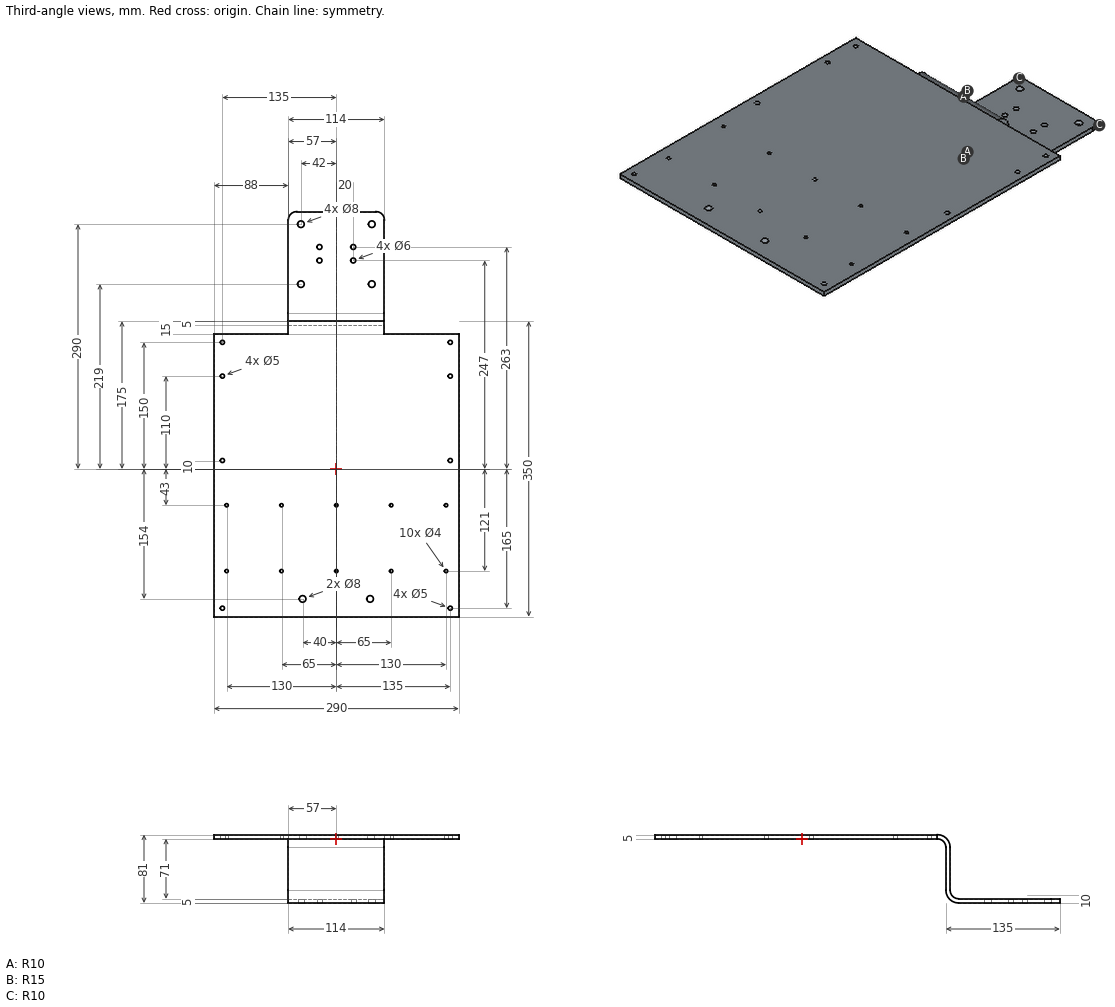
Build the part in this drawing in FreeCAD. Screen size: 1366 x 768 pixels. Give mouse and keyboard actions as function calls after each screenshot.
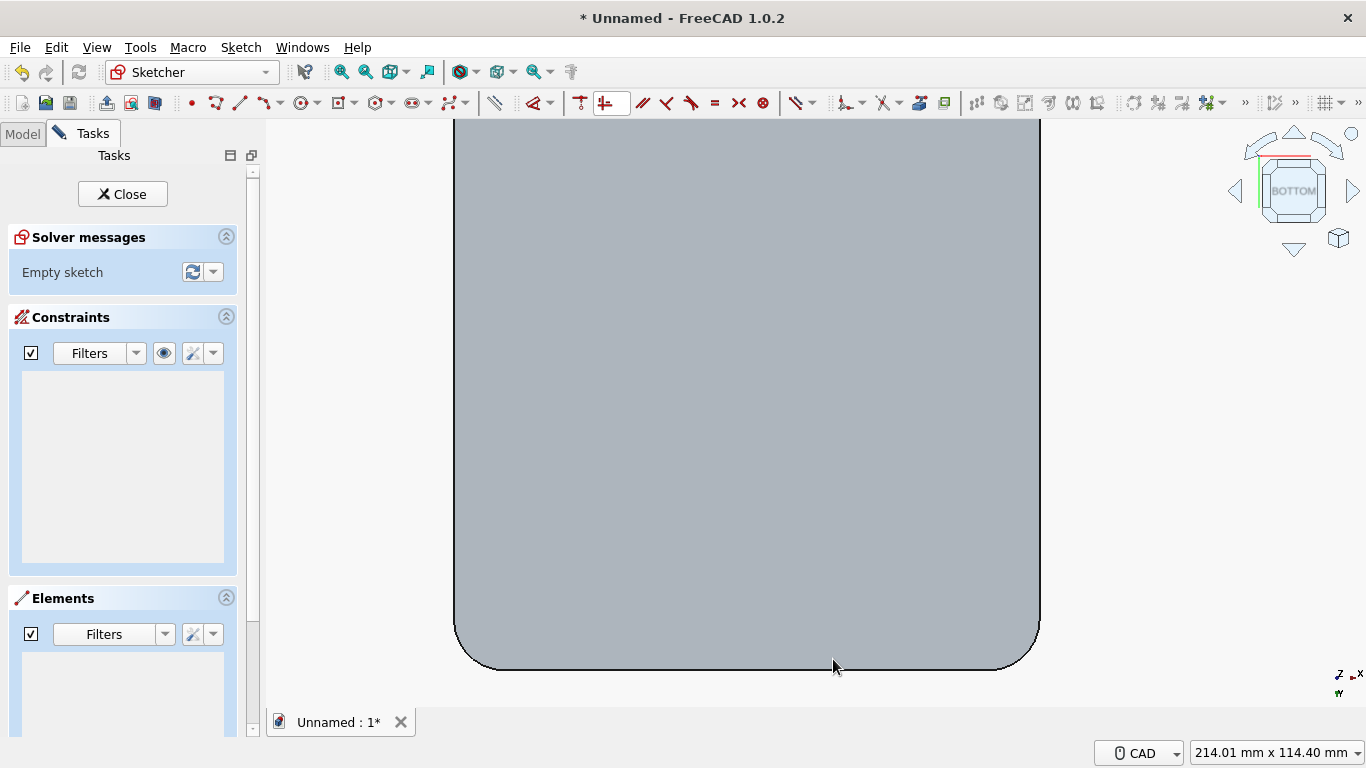
click(302, 104)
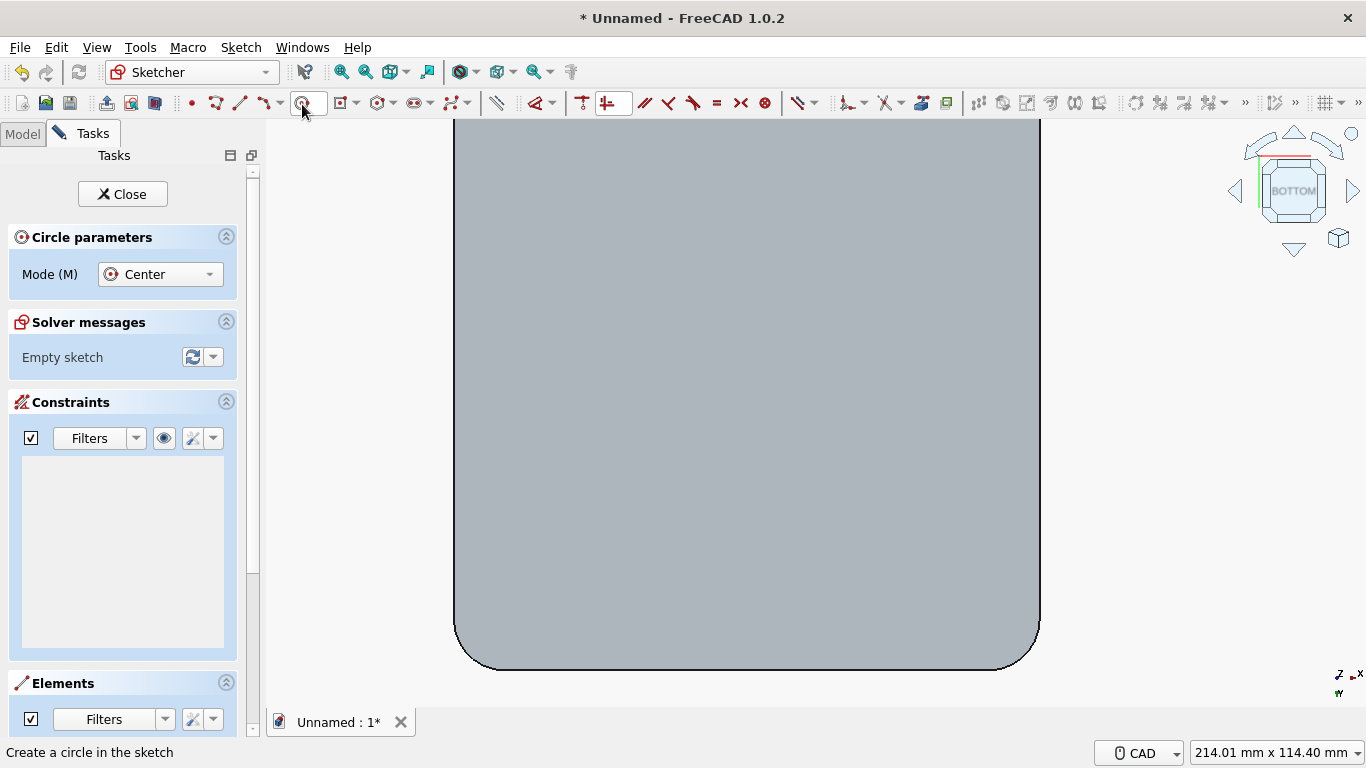
click(531, 593)
click(545, 579)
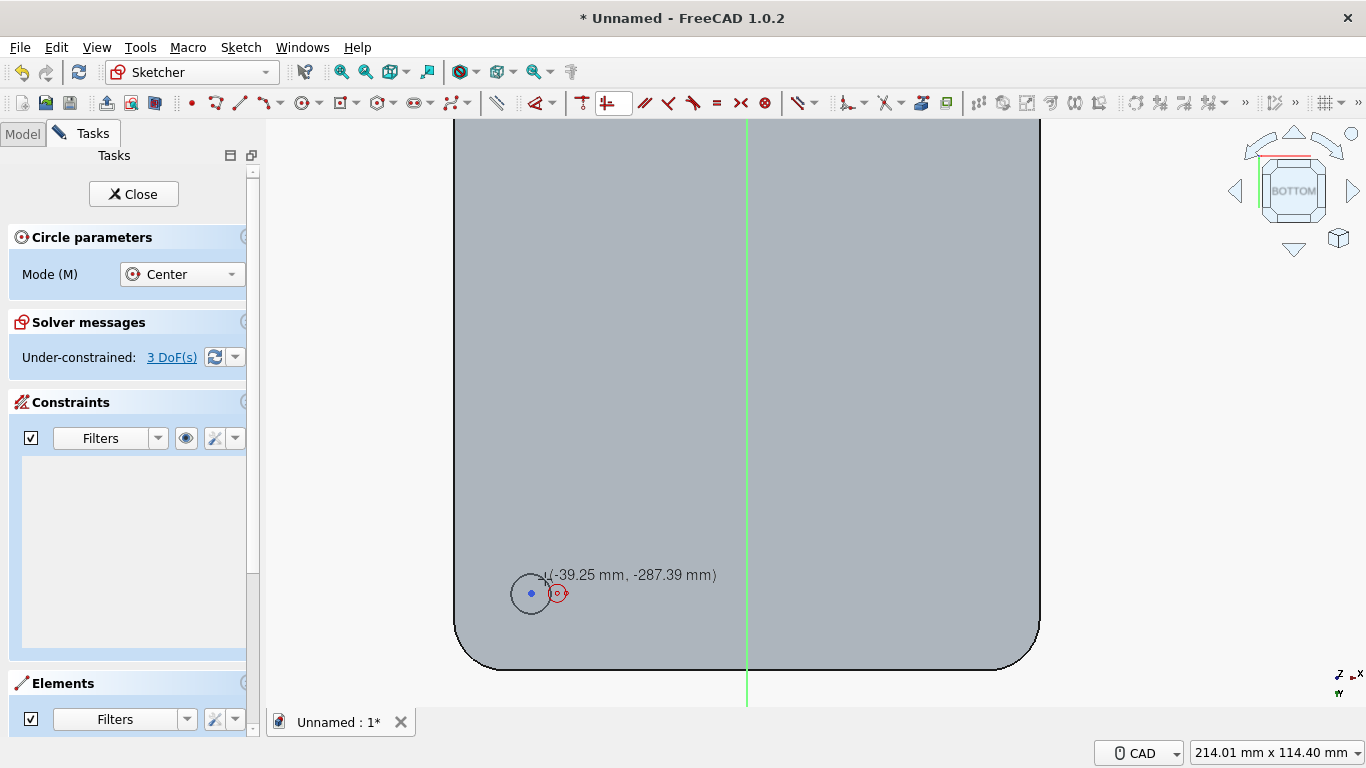
click(963, 593)
click(977, 579)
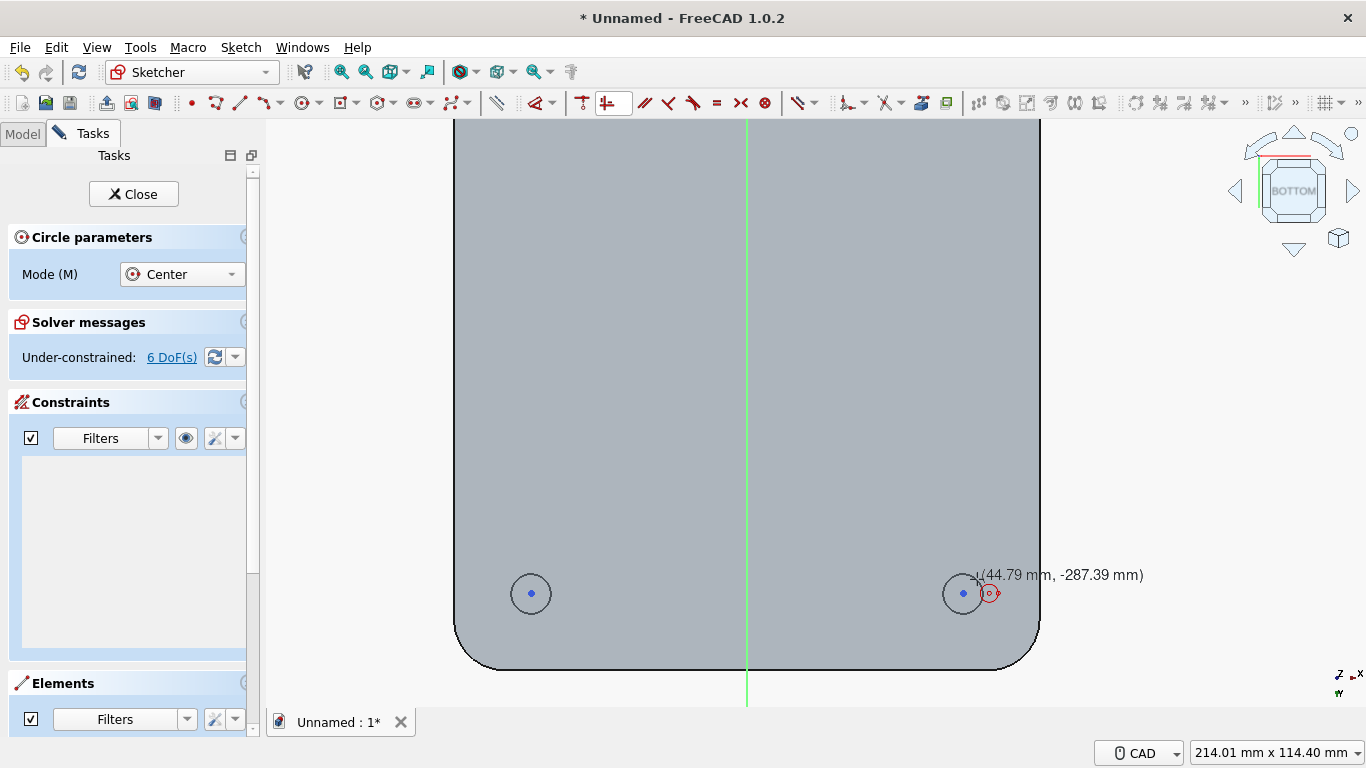
click(531, 228)
click(545, 214)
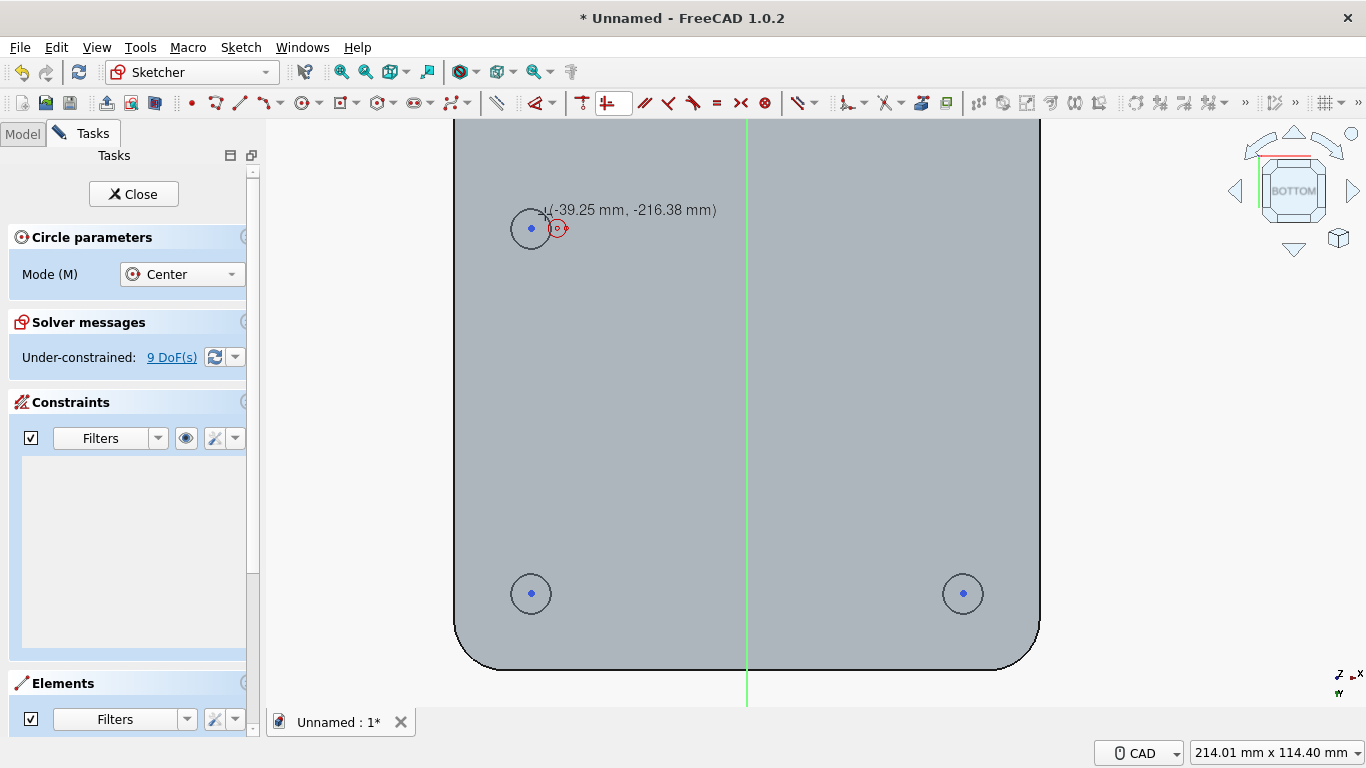
click(963, 228)
click(977, 214)
key(Escape)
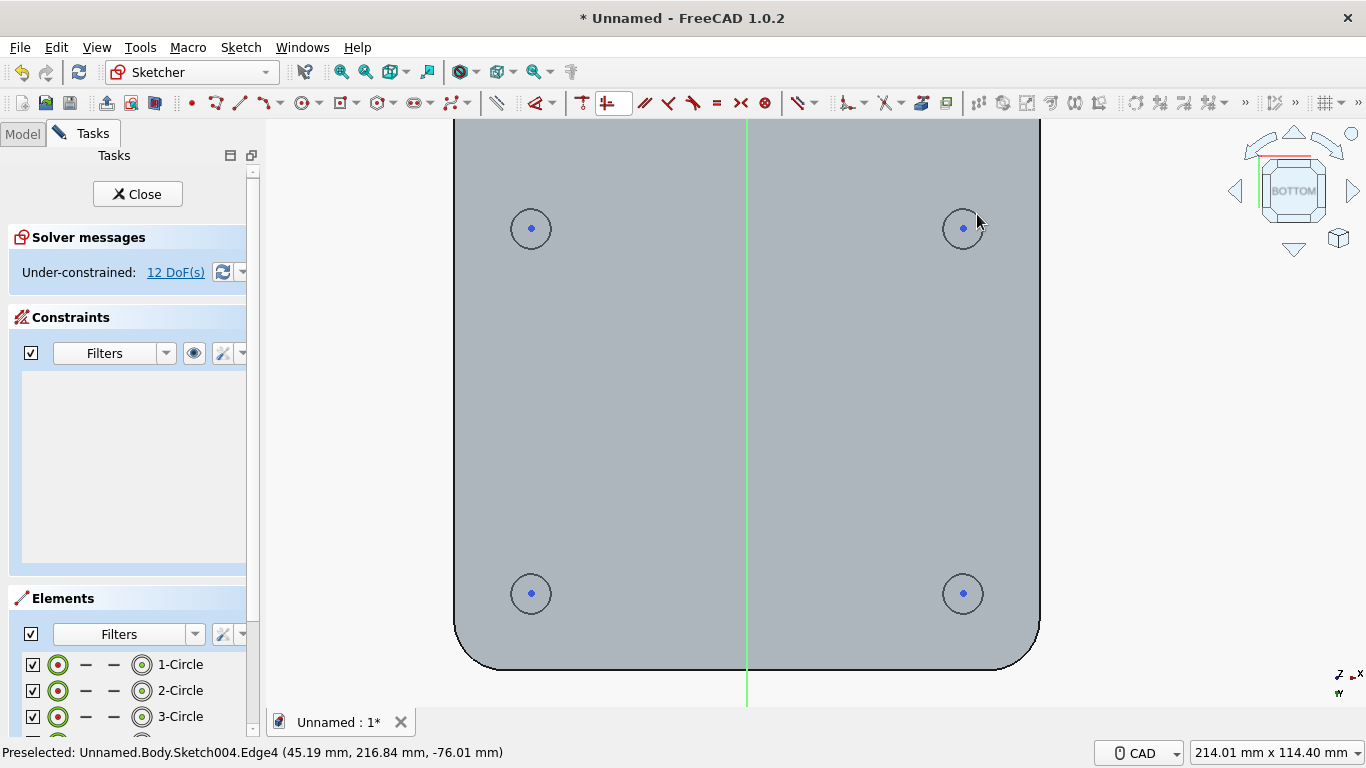
click(545, 580)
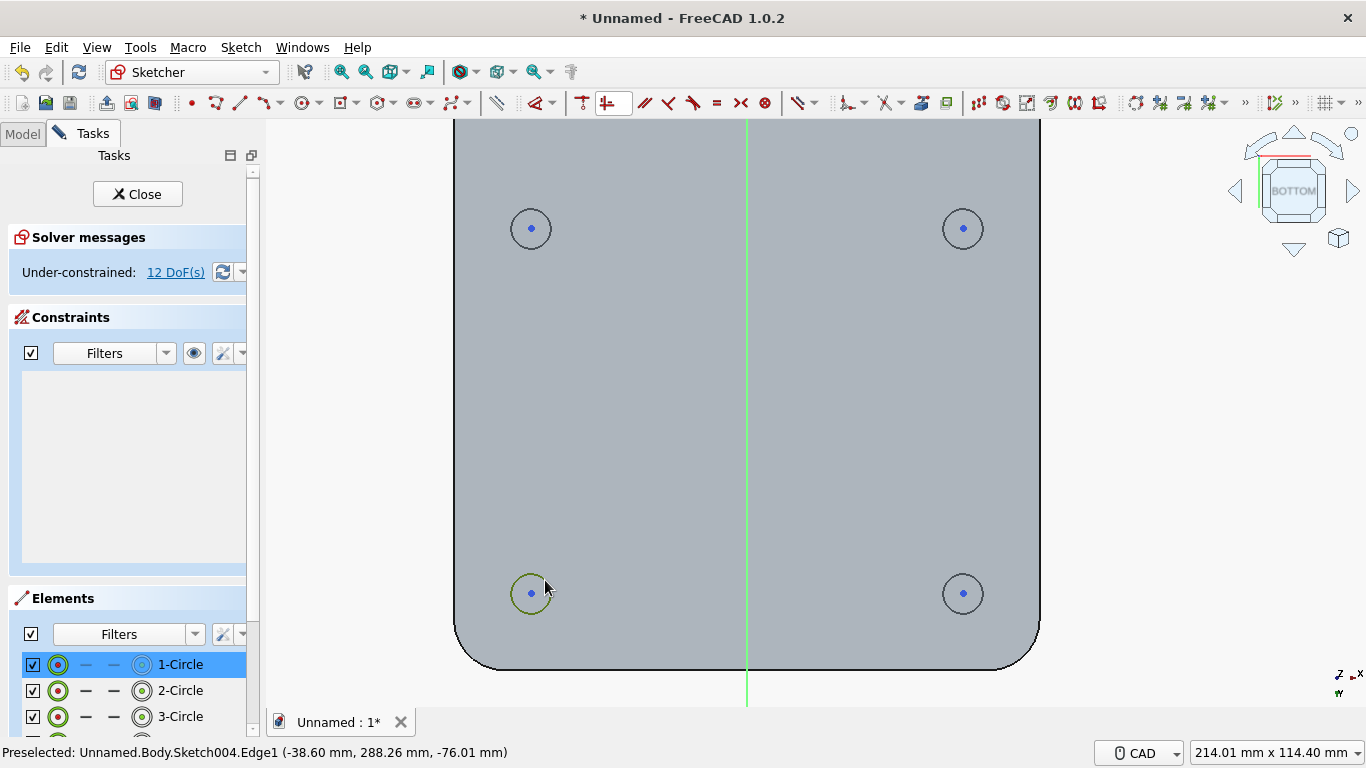
click(977, 580)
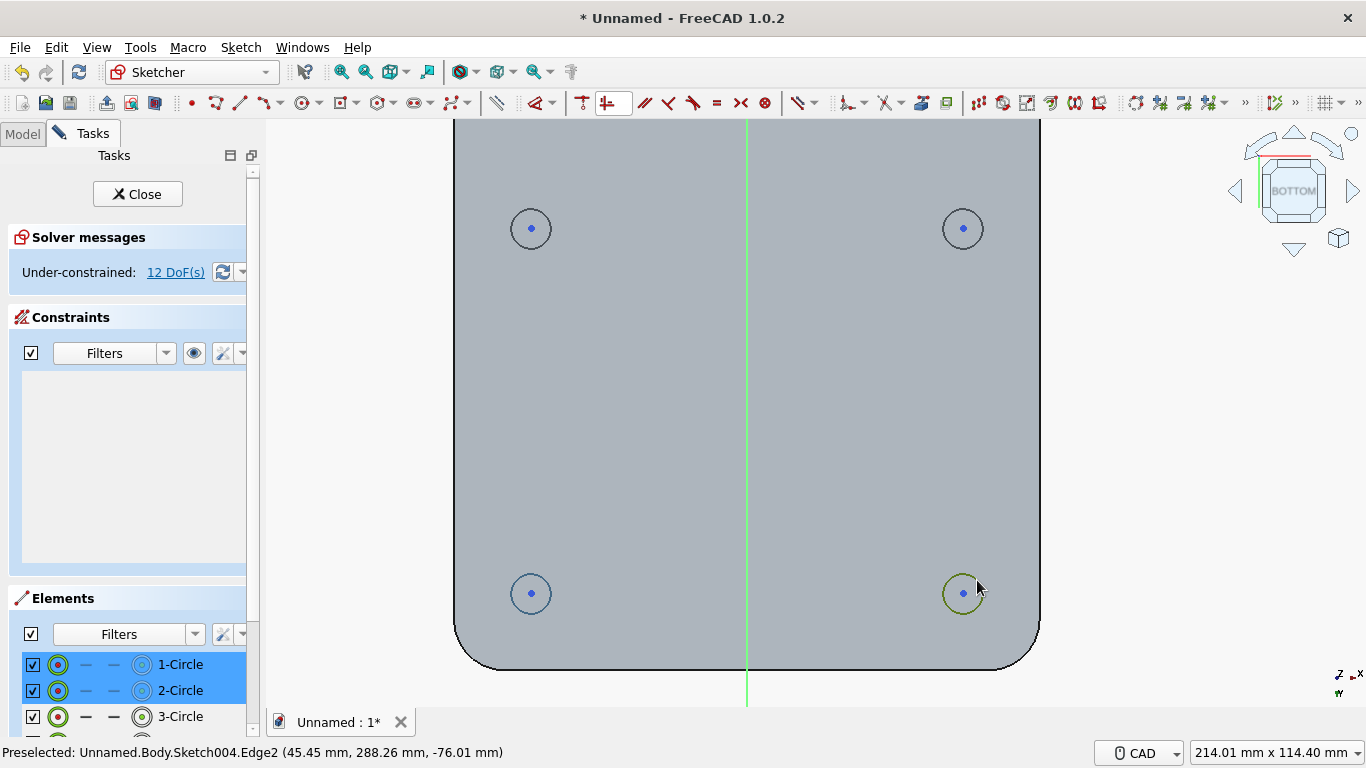
click(545, 215)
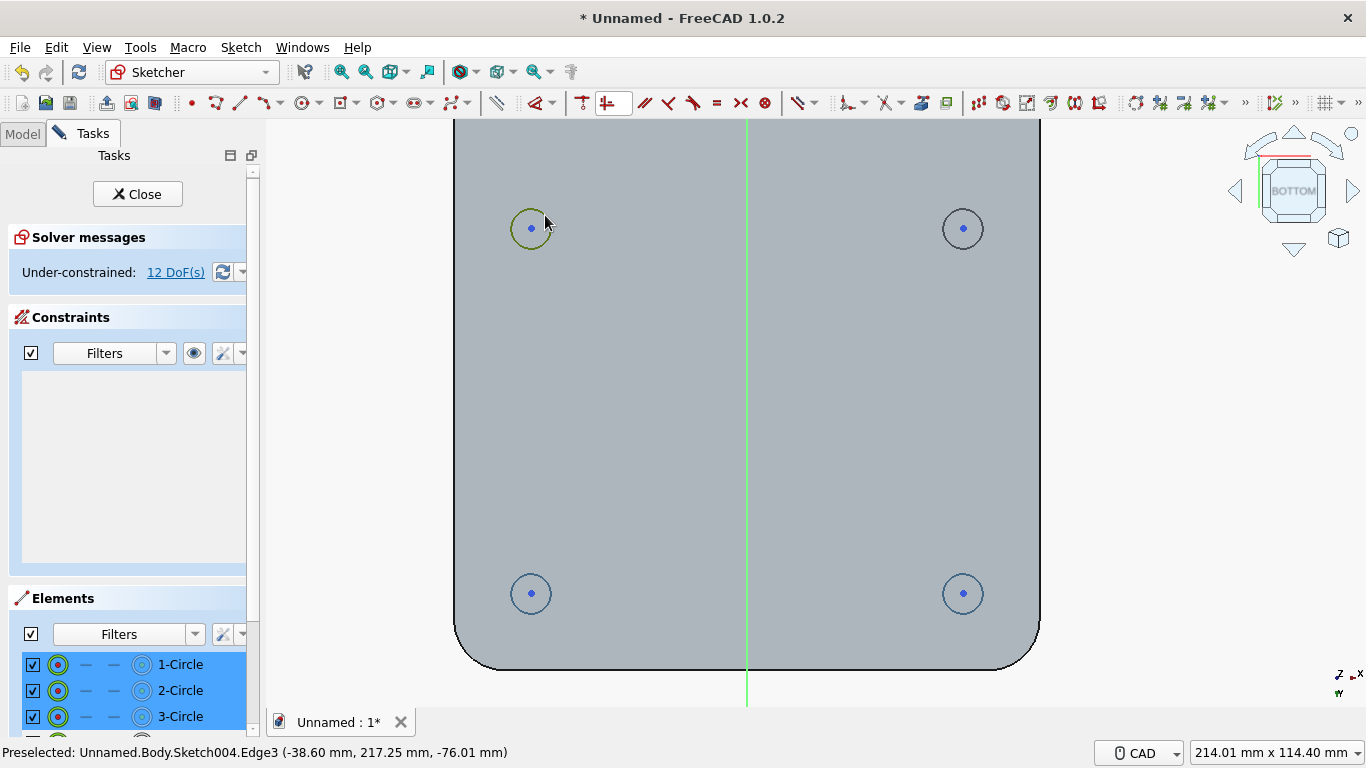
click(977, 215)